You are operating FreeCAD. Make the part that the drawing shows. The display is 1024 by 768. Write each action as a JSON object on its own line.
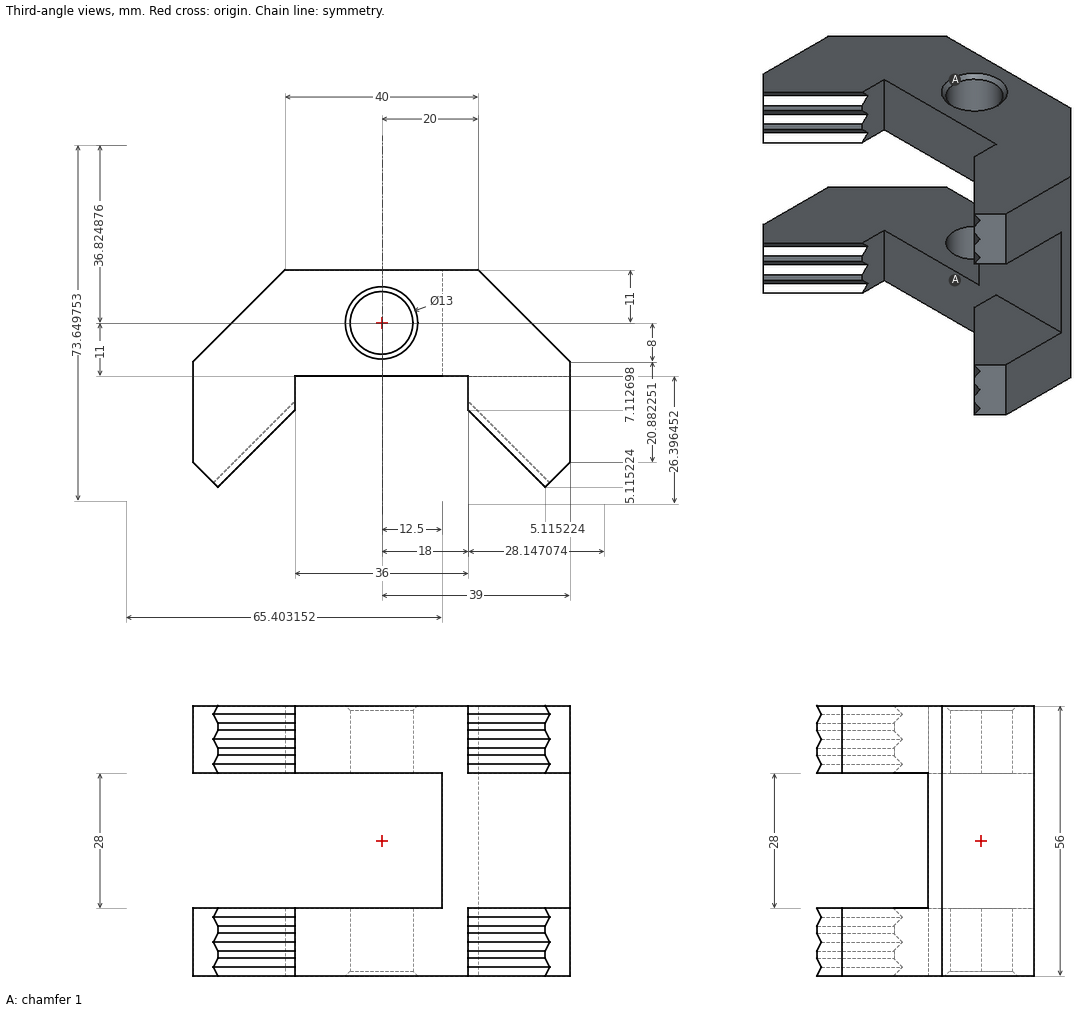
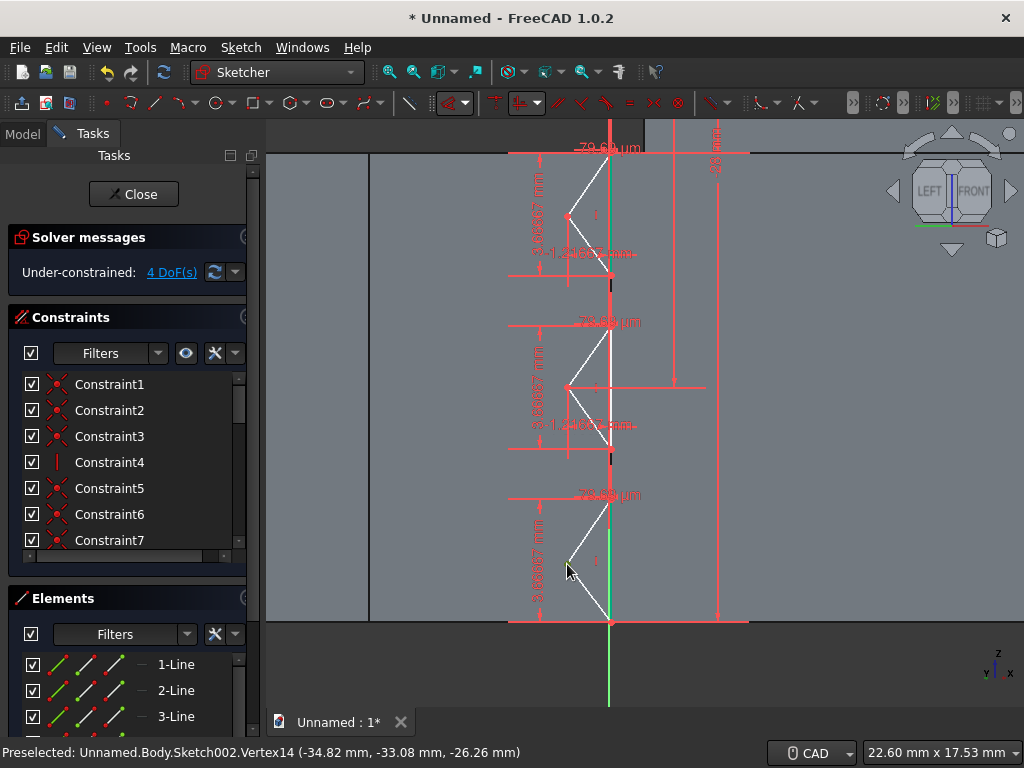
{"action": "key", "text": "l"}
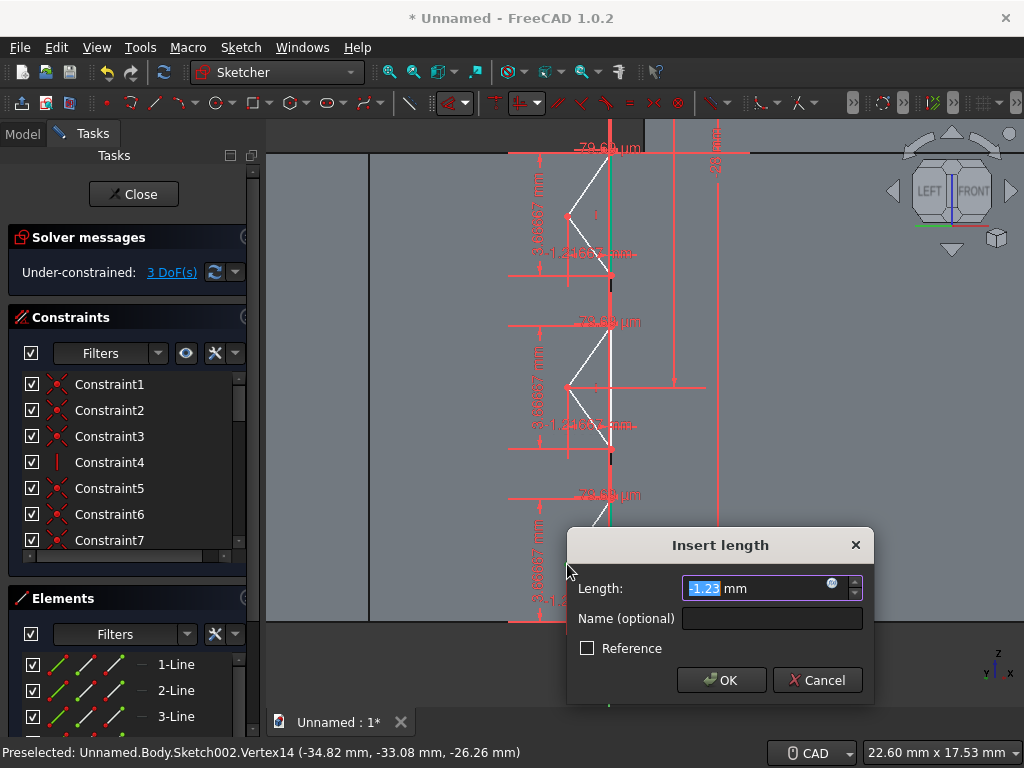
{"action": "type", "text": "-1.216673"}
{"action": "key", "text": "Return"}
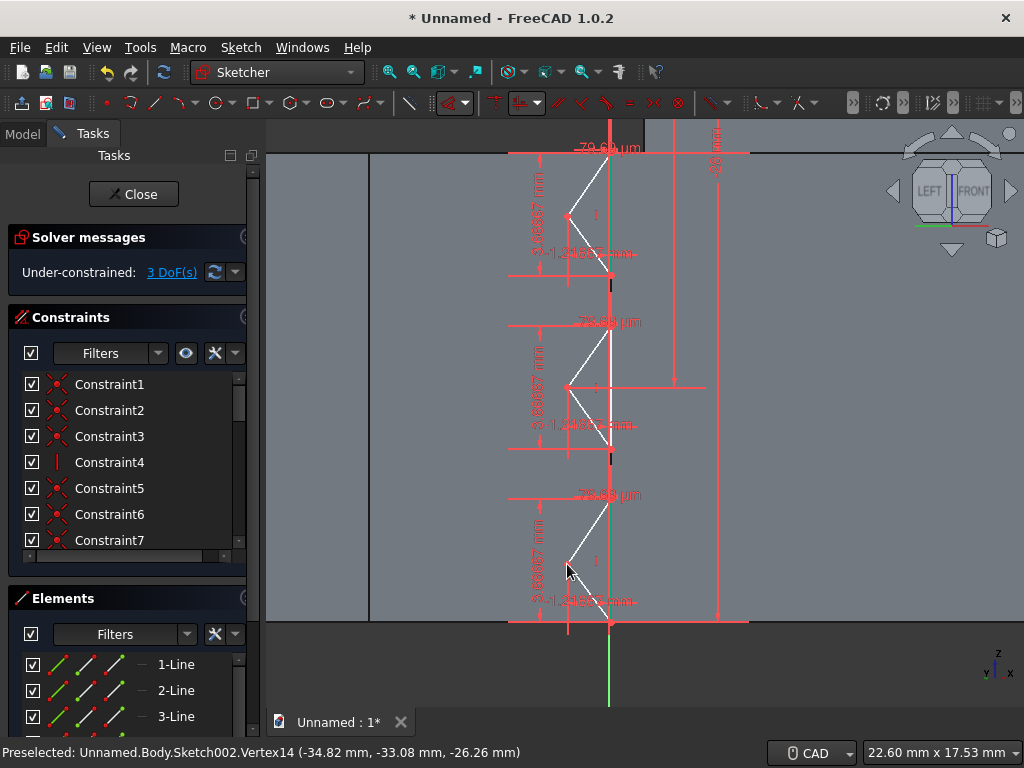
{"action": "scroll", "coordinate": [598, 345], "scroll_direction": "up", "scroll_amount": 2}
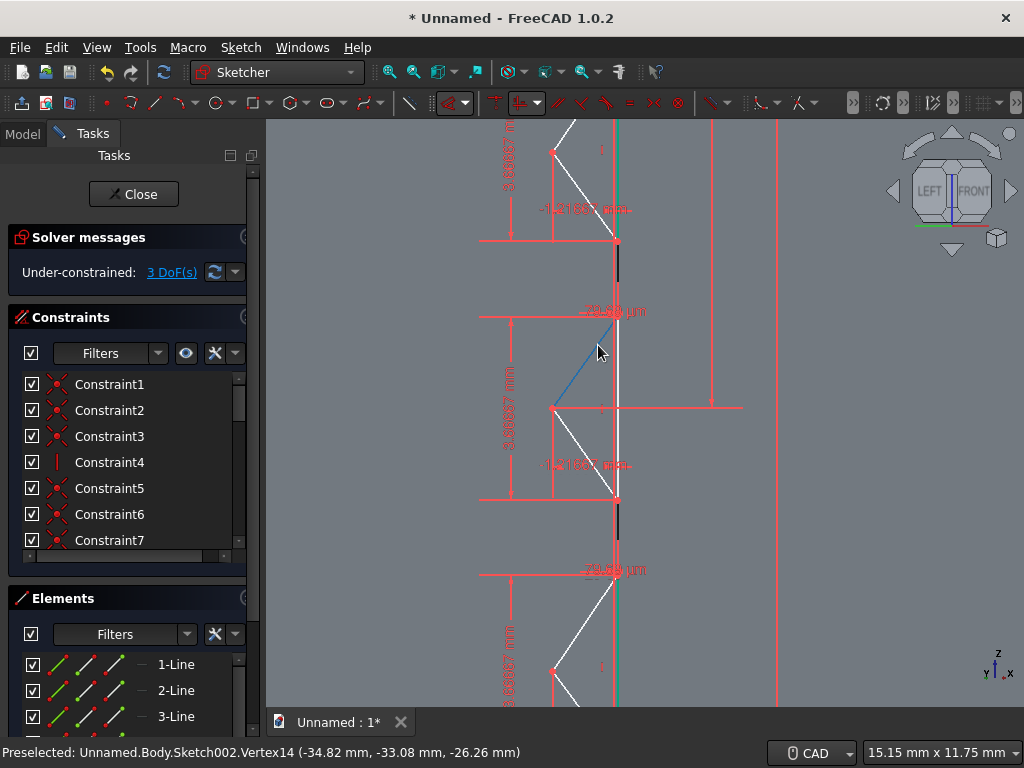
{"action": "left_click", "coordinate": [598, 344]}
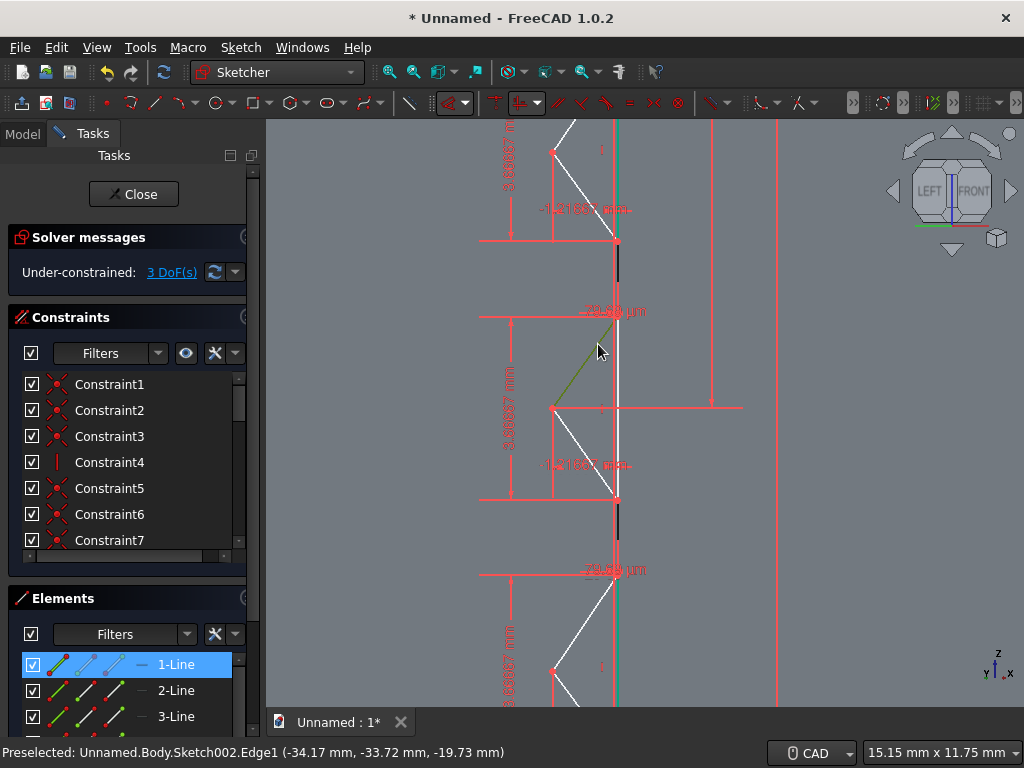
{"action": "key", "text": "i"}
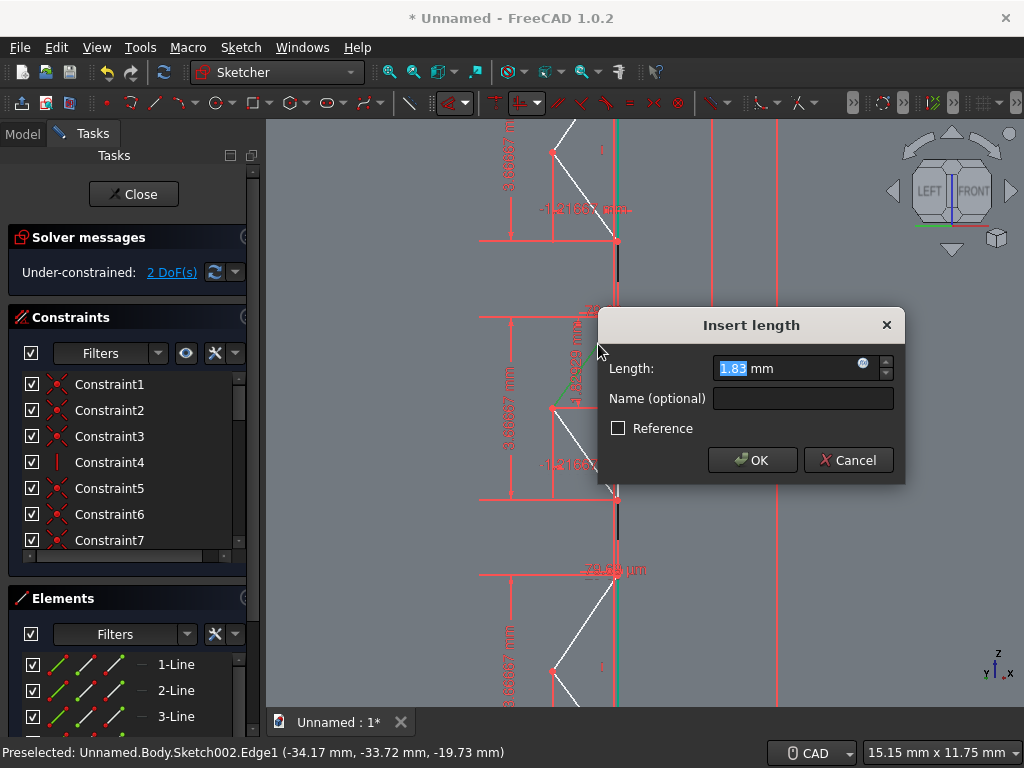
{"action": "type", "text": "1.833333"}
{"action": "key", "text": "Return"}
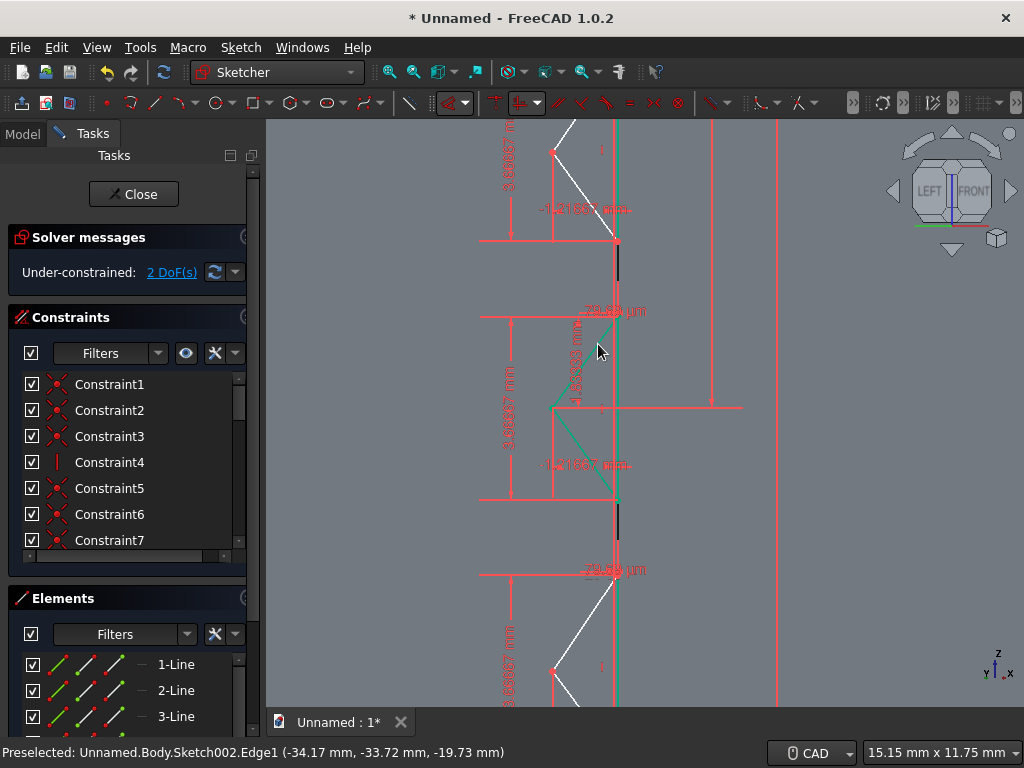
{"action": "scroll", "coordinate": [574, 529], "scroll_direction": "down", "scroll_amount": 7}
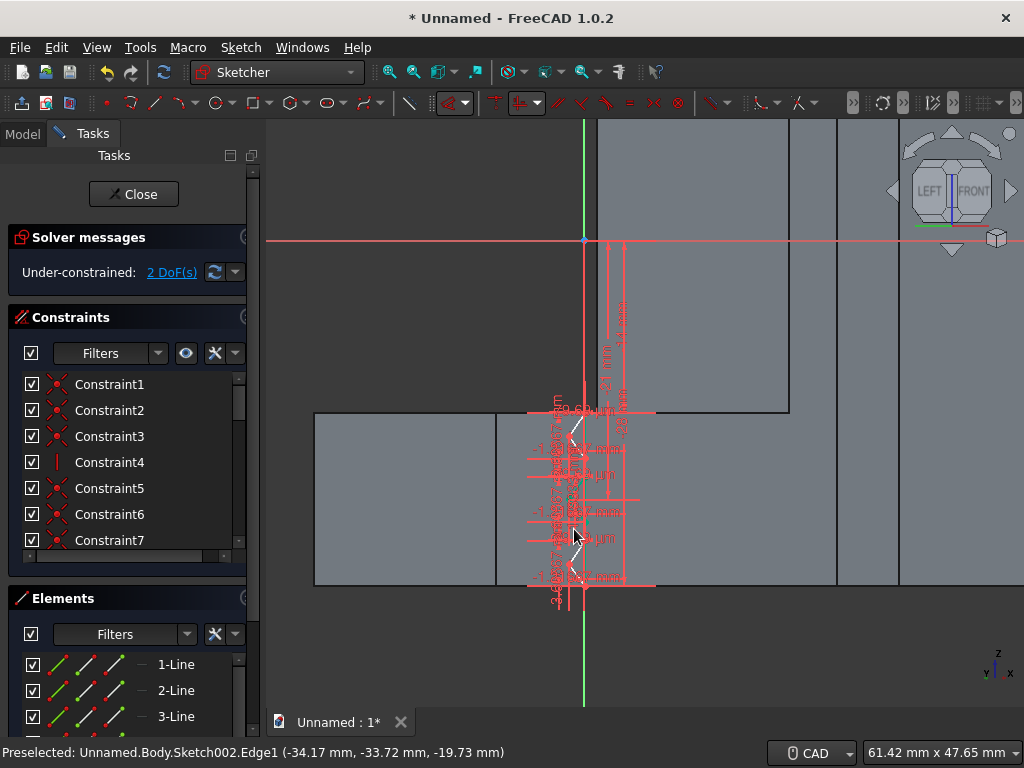
{"action": "scroll", "coordinate": [580, 420], "scroll_direction": "up", "scroll_amount": 7}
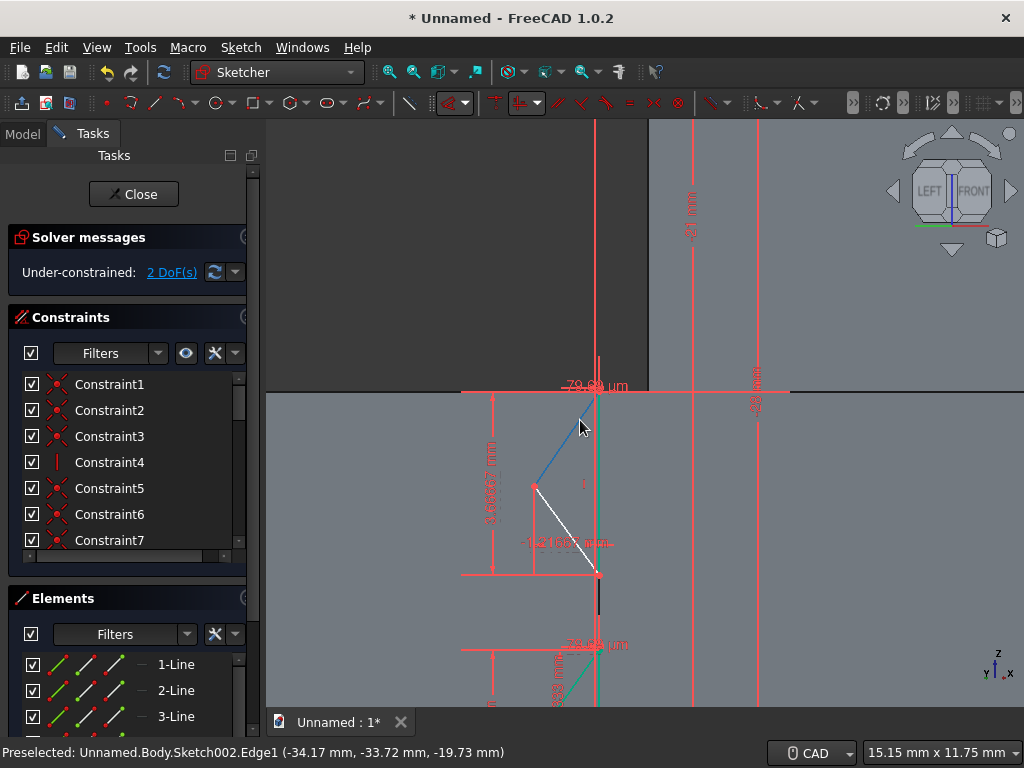
{"action": "left_click", "coordinate": [580, 420]}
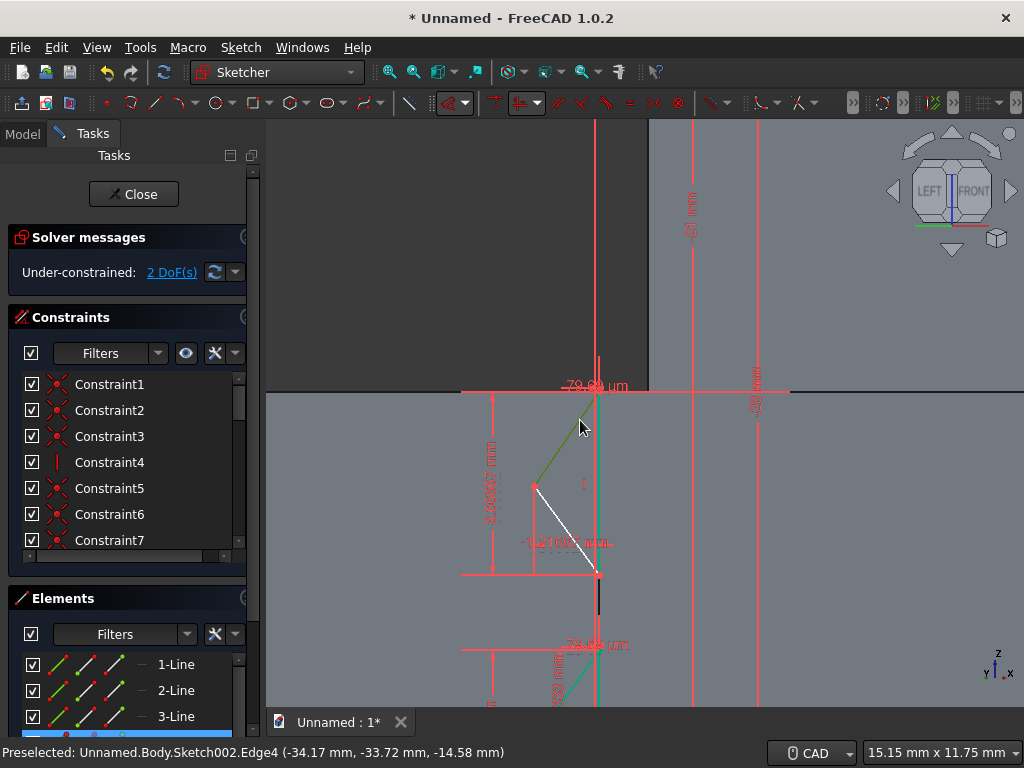
{"action": "key", "text": "i"}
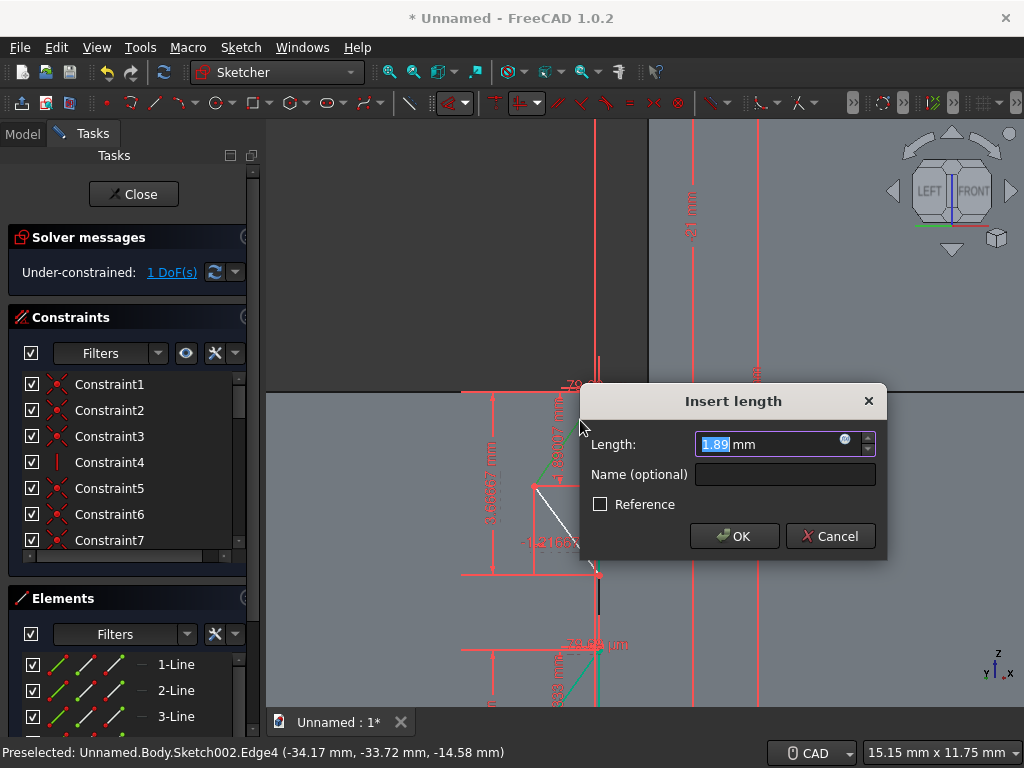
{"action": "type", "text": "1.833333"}
{"action": "key", "text": "Return"}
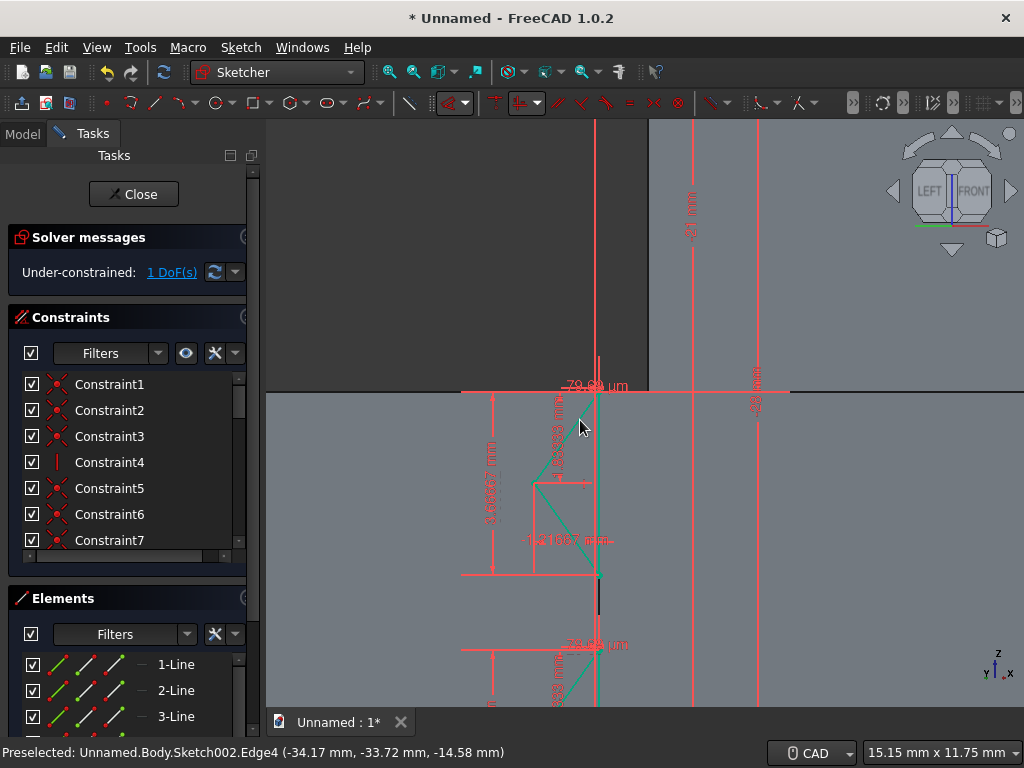
{"action": "scroll", "coordinate": [580, 420], "scroll_direction": "down", "scroll_amount": 7}